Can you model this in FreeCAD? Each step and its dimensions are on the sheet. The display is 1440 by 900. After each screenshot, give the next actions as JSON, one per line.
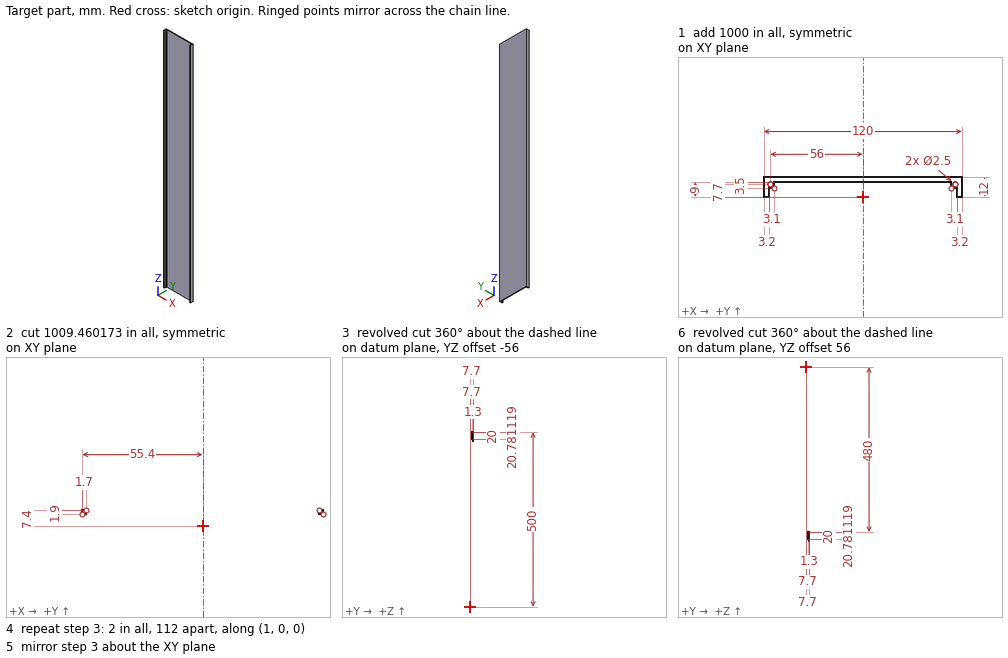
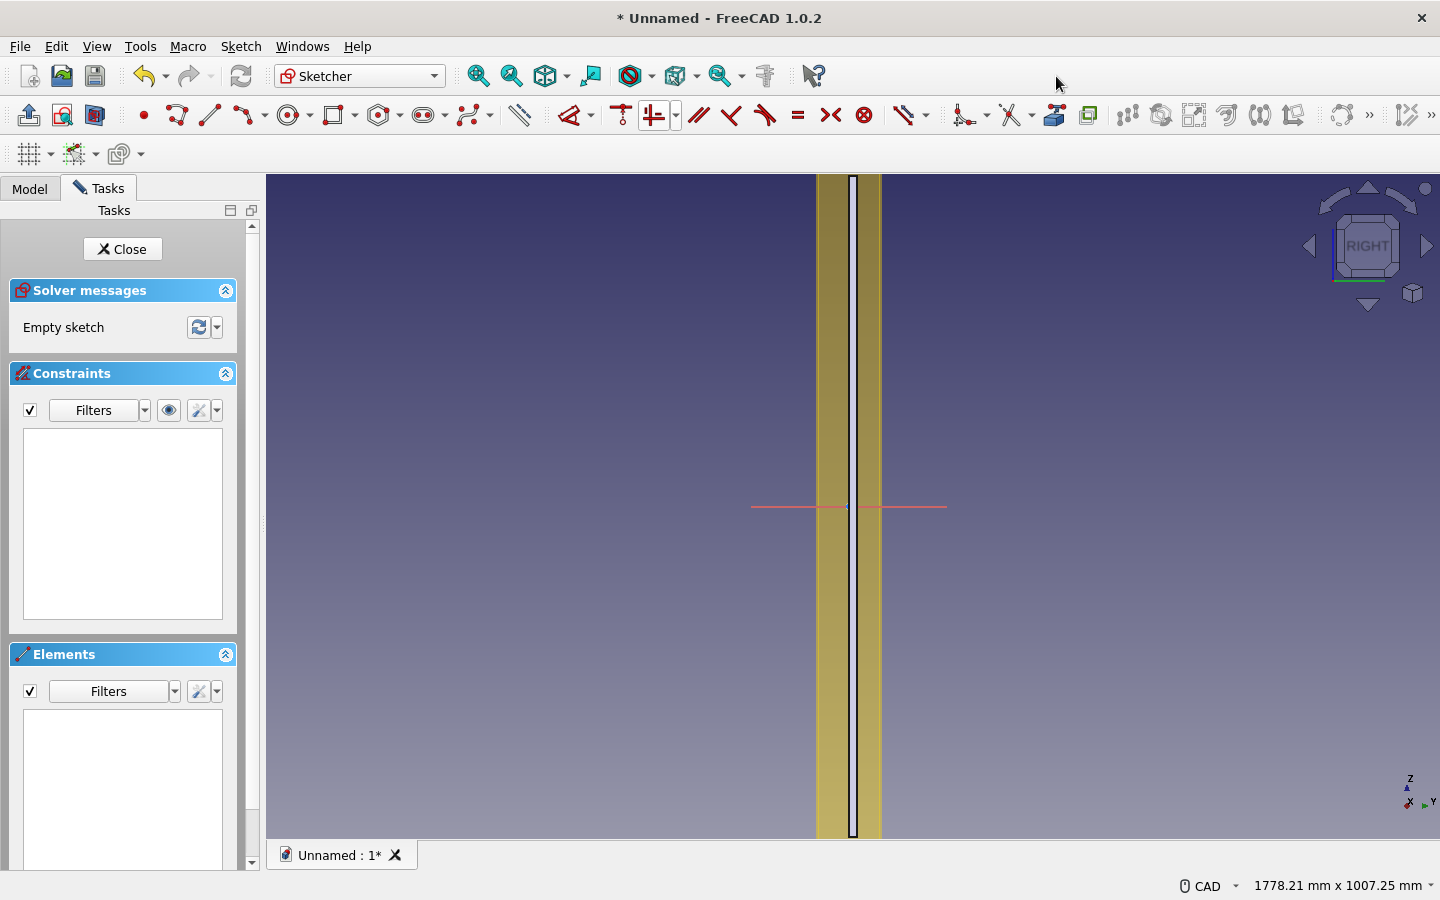
{"action": "key", "text": "q s"}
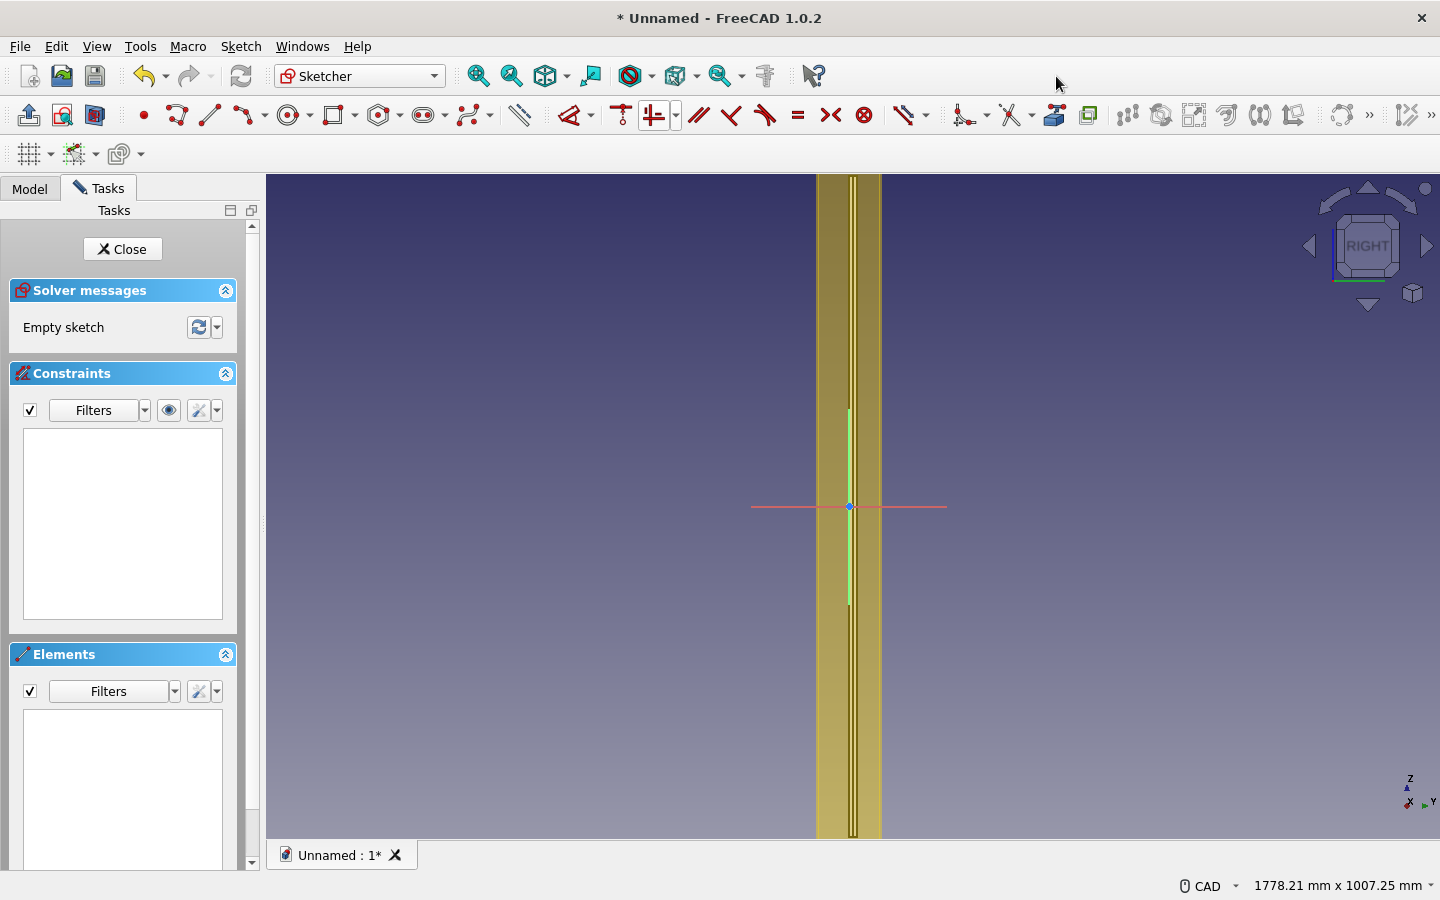
{"action": "scroll", "coordinate": [784, 506], "scroll_direction": "down", "scroll_amount": 5}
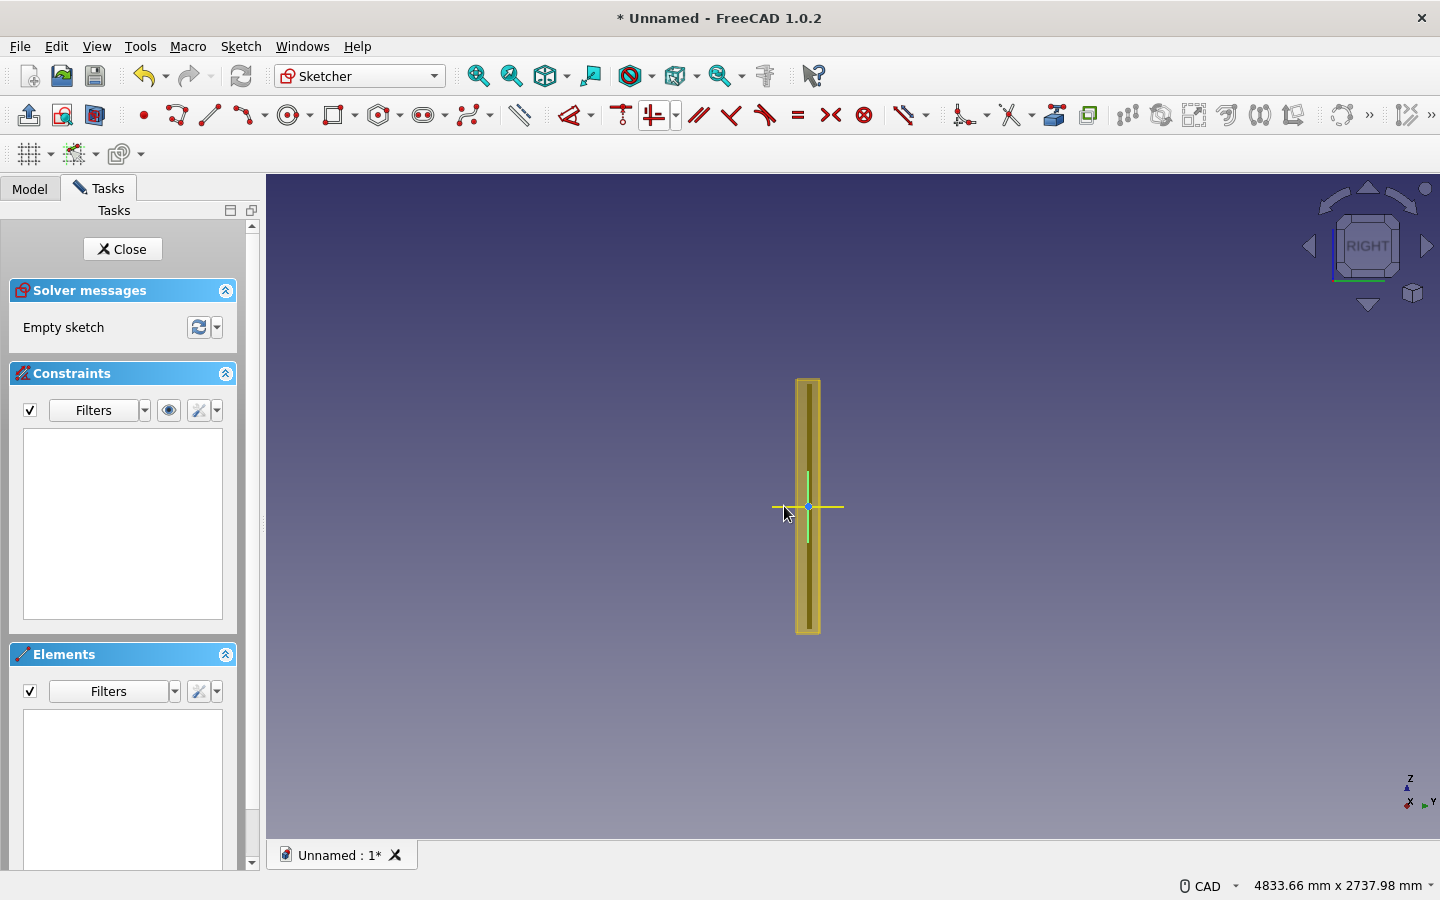
{"action": "scroll", "coordinate": [811, 382], "scroll_direction": "up", "scroll_amount": 15}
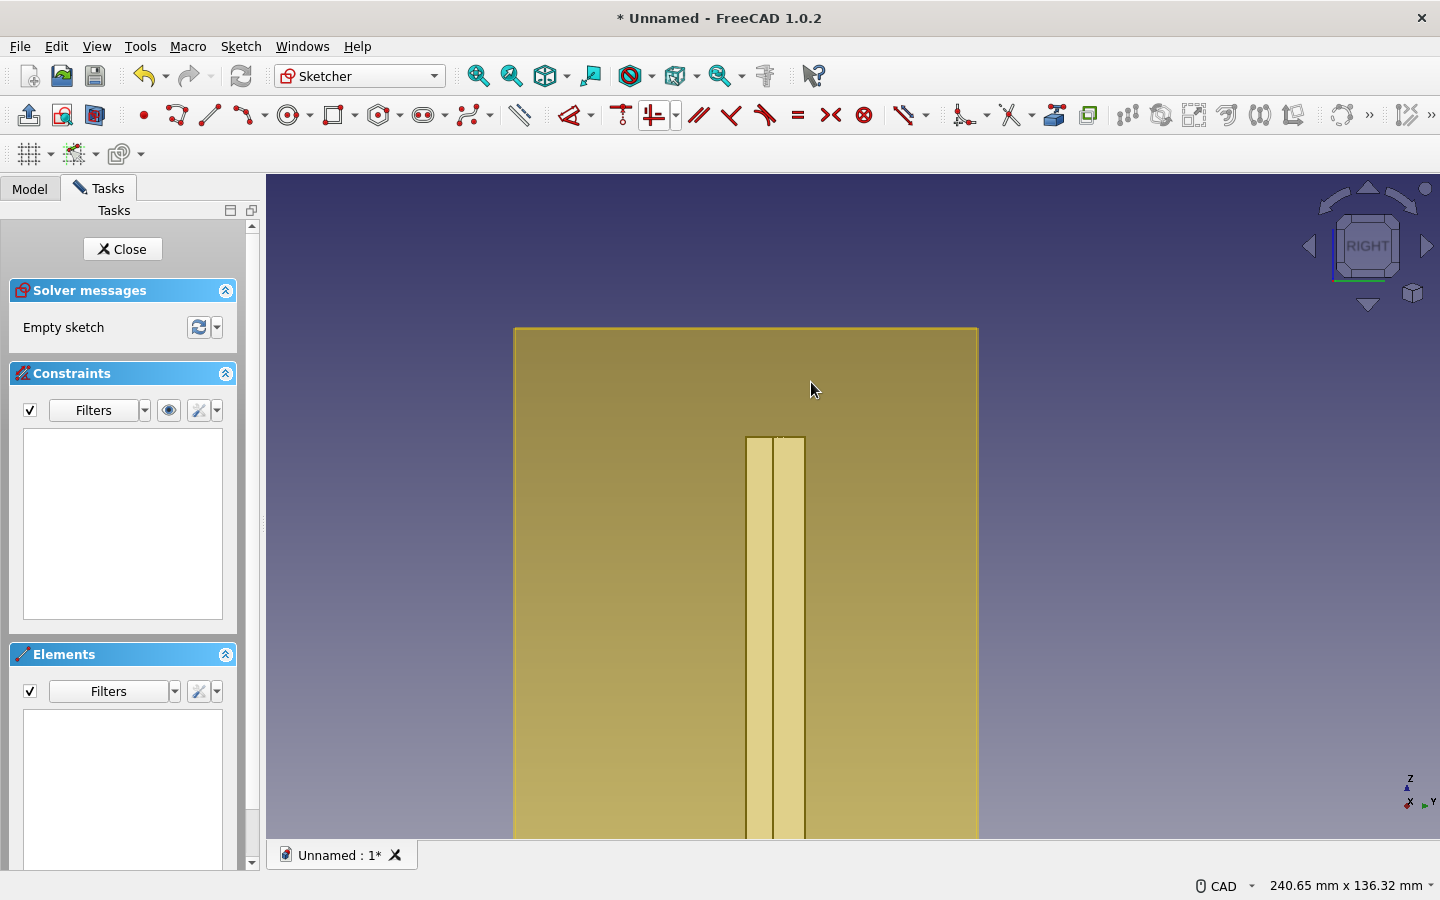
{"action": "scroll", "coordinate": [779, 509], "scroll_direction": "up", "scroll_amount": 6}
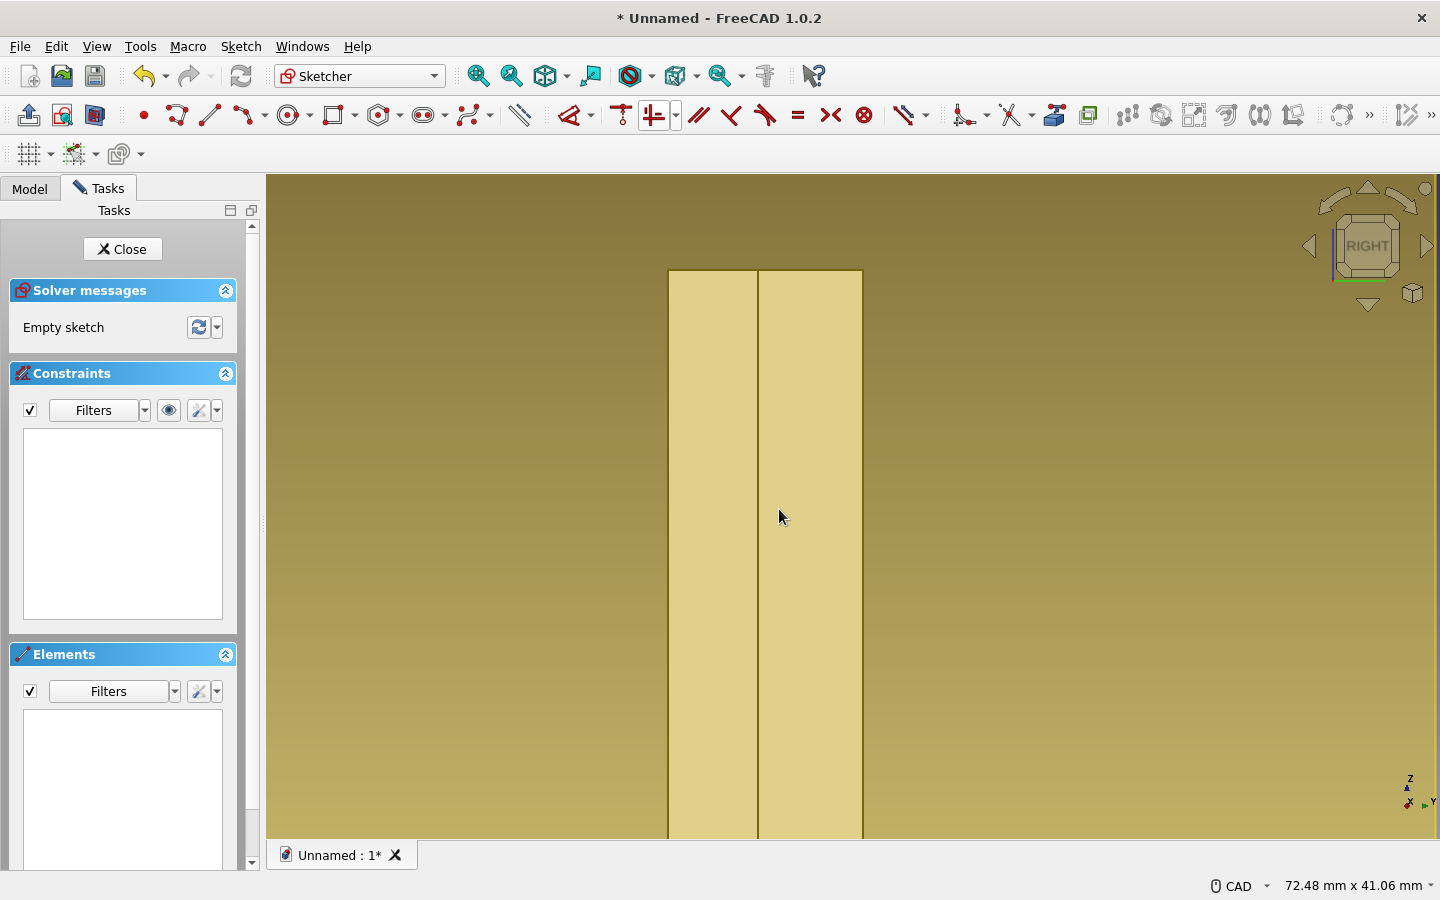
{"action": "key", "text": "g m"}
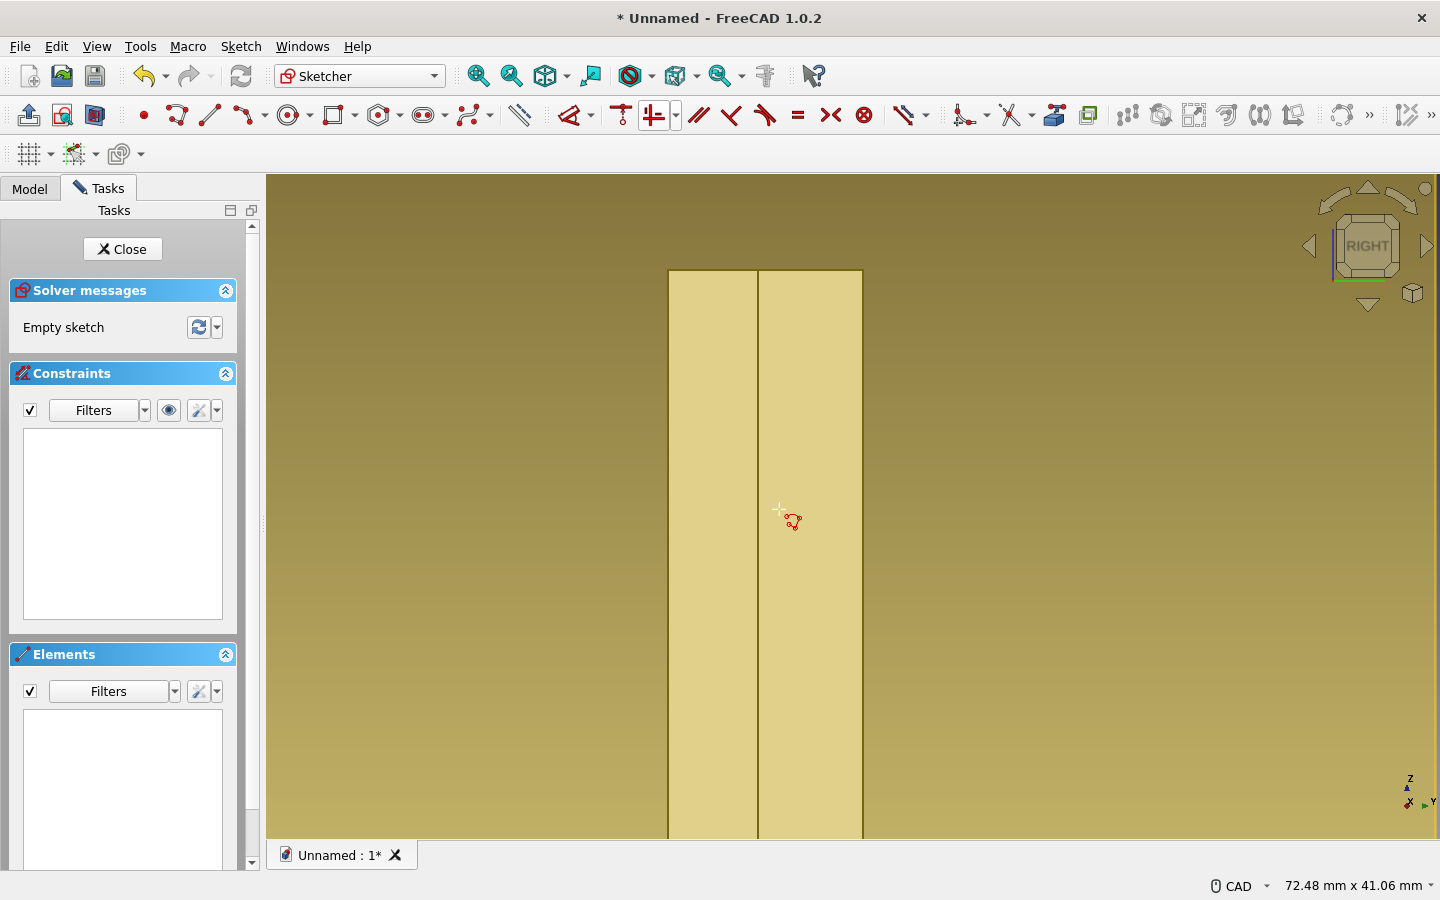
{"action": "left_click", "coordinate": [793, 607]}
{"action": "left_click", "coordinate": [793, 270]}
{"action": "left_click", "coordinate": [772, 270]}
{"action": "left_click", "coordinate": [772, 594]}
{"action": "left_click", "coordinate": [793, 608]}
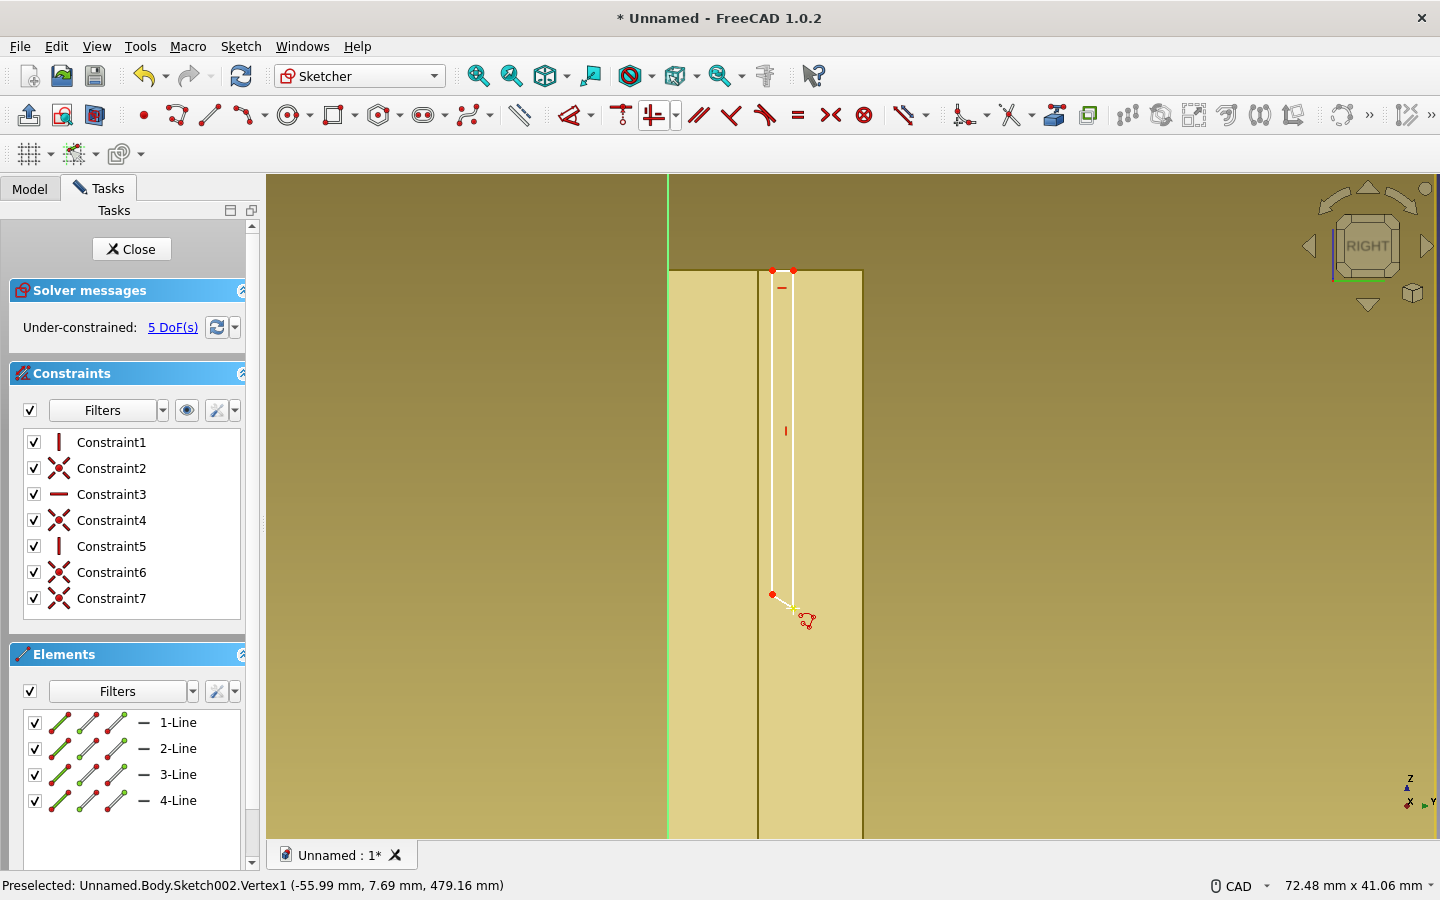
{"action": "left_click", "coordinate": [210, 116]}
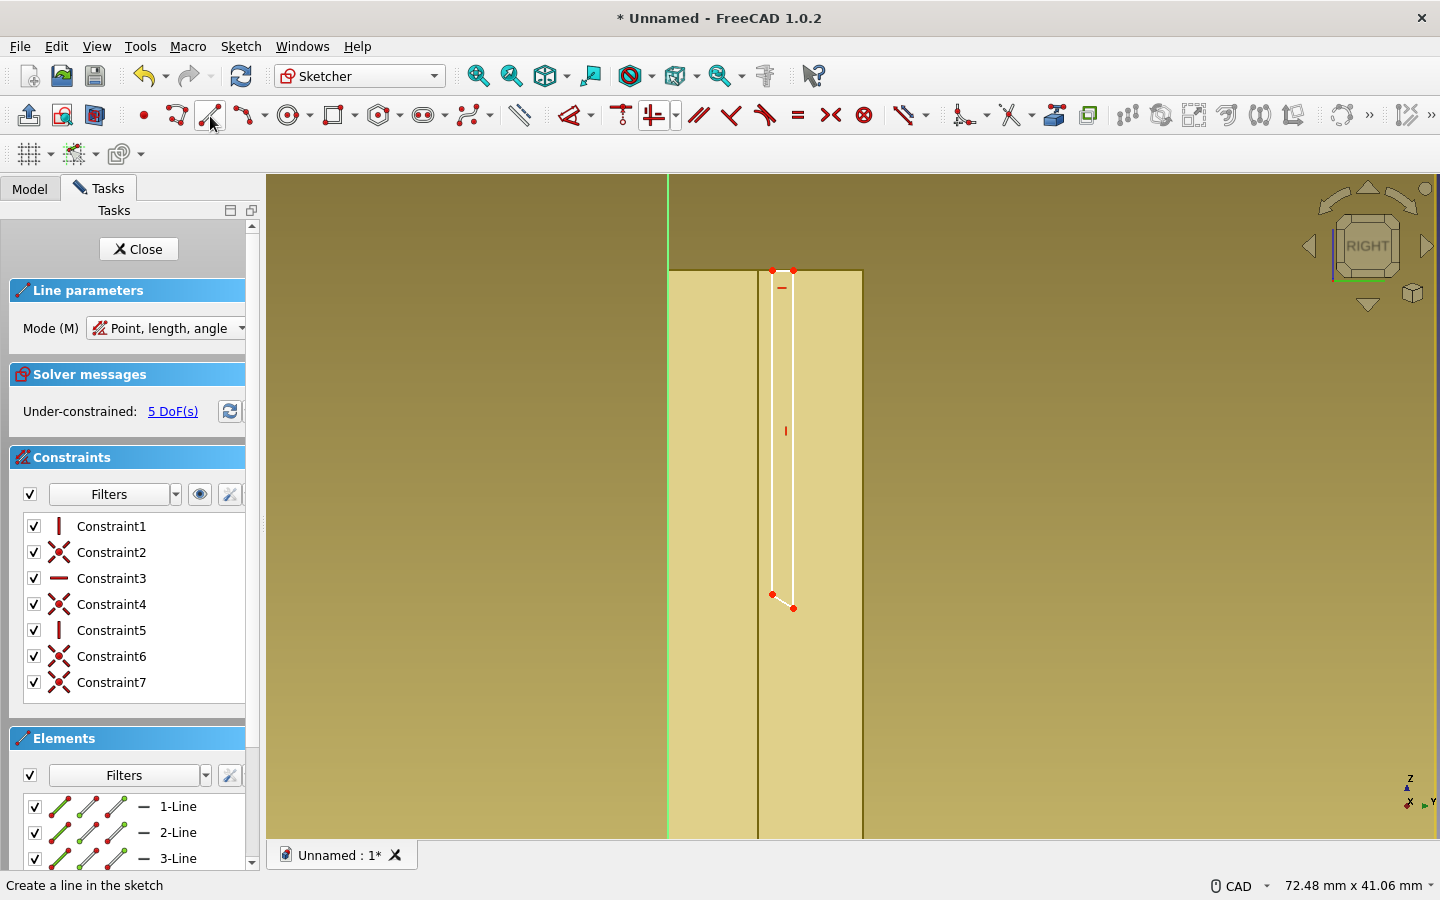
{"action": "left_click", "coordinate": [793, 641]}
{"action": "left_click", "coordinate": [793, 742]}
{"action": "key", "text": "Escape"}